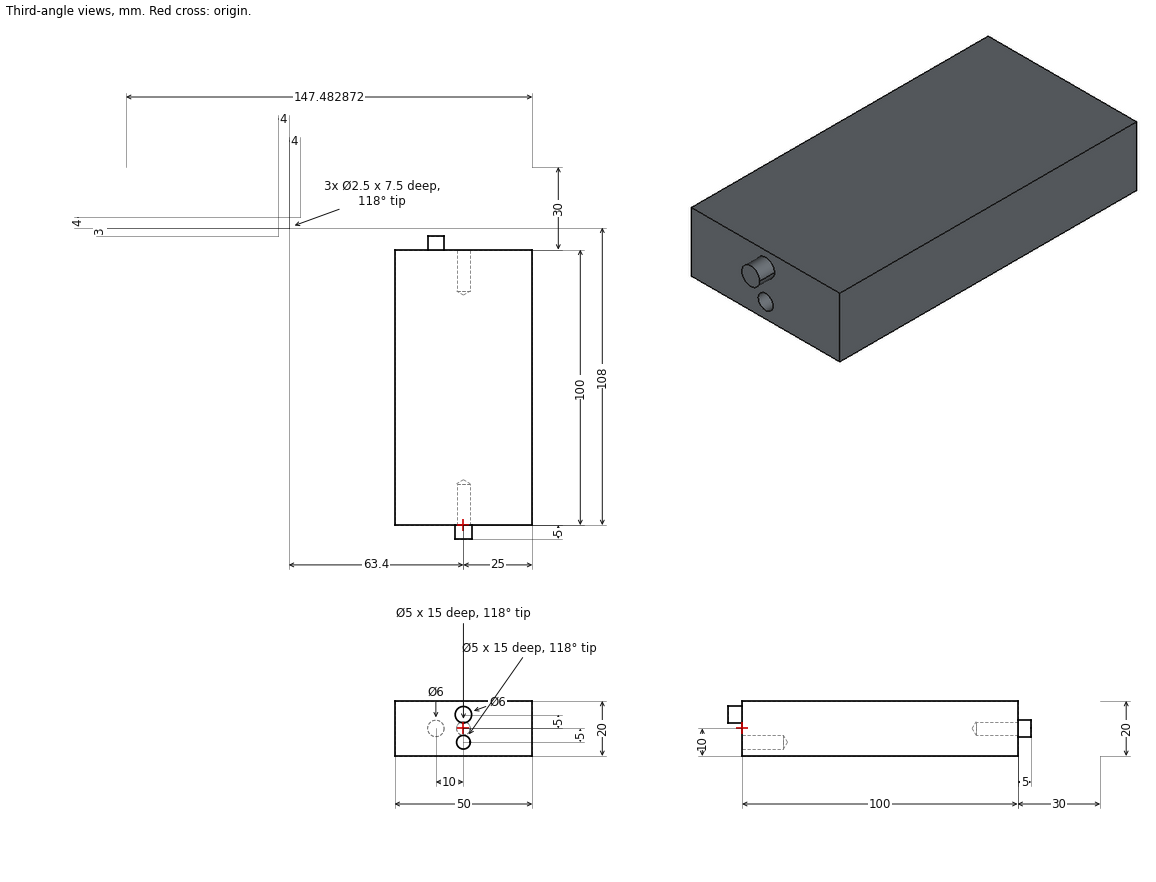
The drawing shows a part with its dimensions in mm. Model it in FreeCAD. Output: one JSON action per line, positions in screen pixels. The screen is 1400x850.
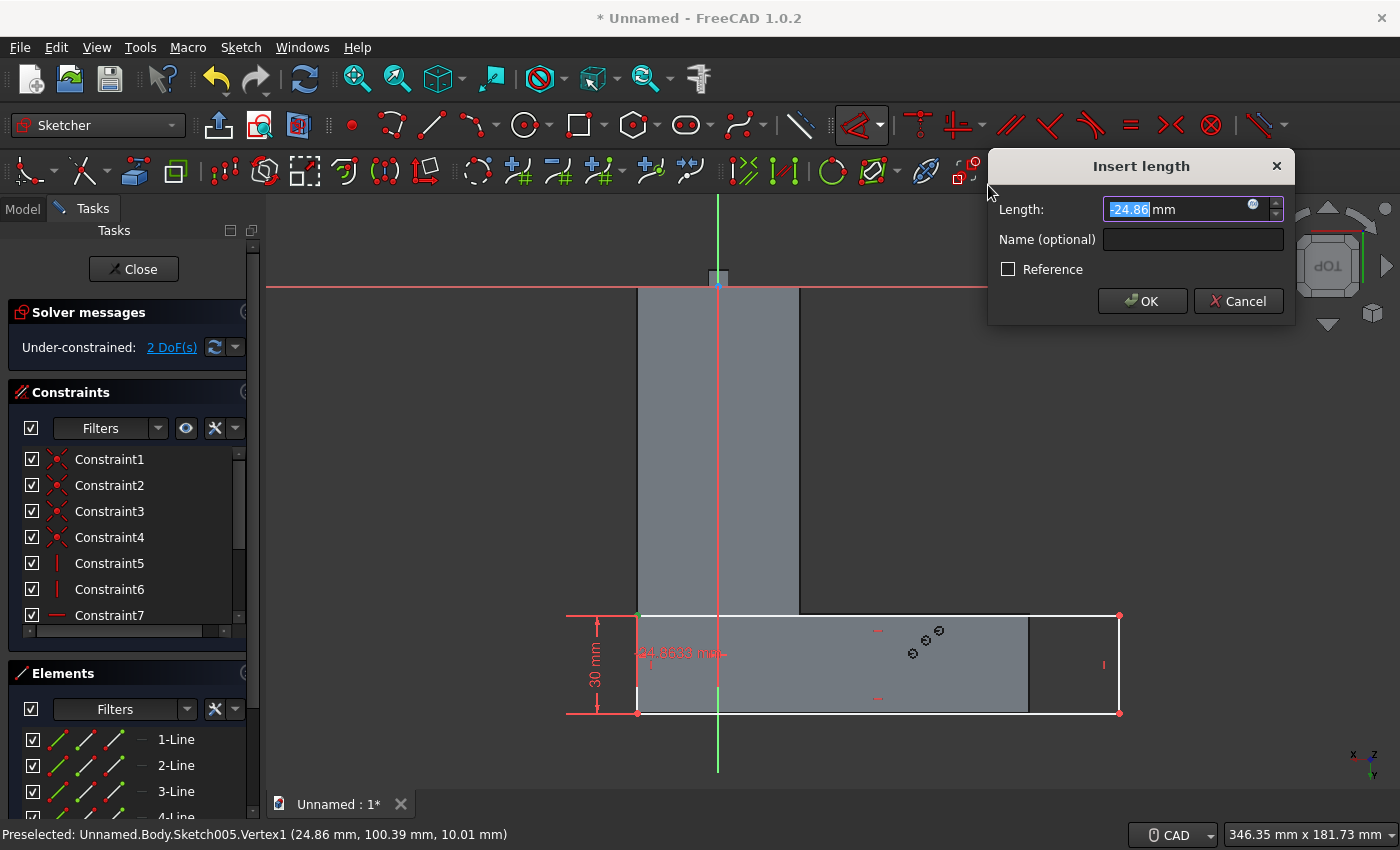
{"action": "type", "text": "-25"}
{"action": "key", "text": "Return"}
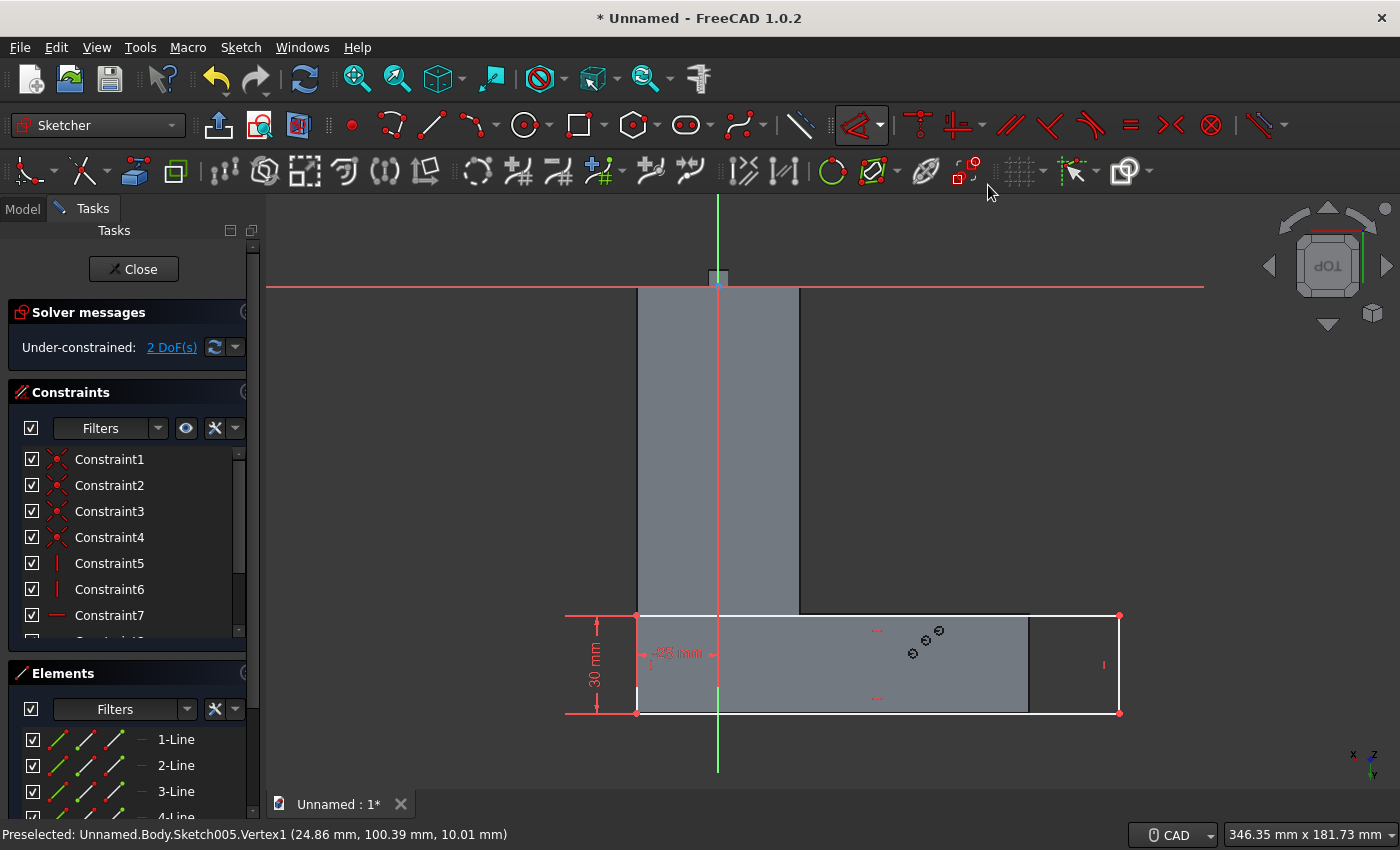
{"action": "left_click", "coordinate": [637, 616]}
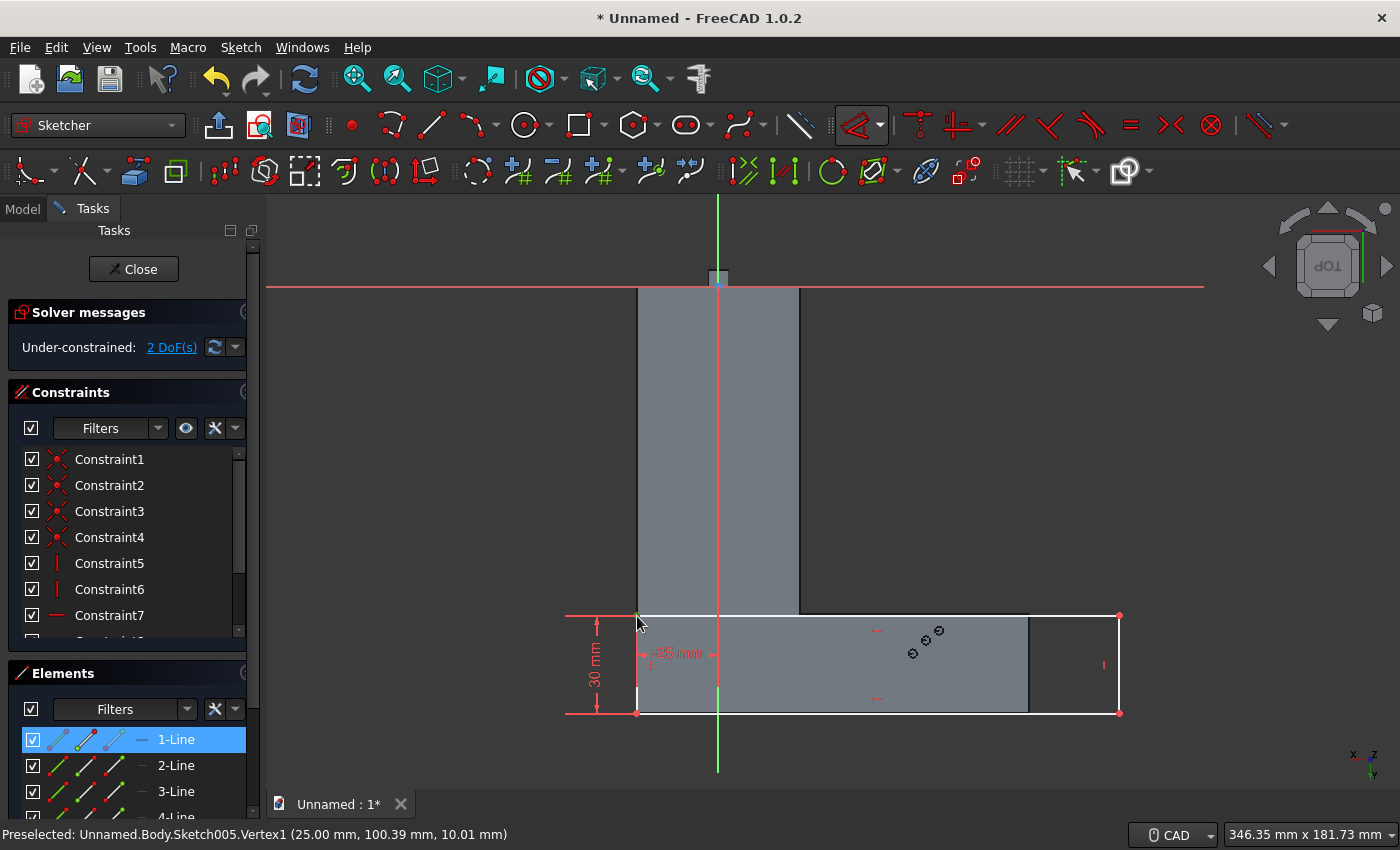
{"action": "key", "text": "i"}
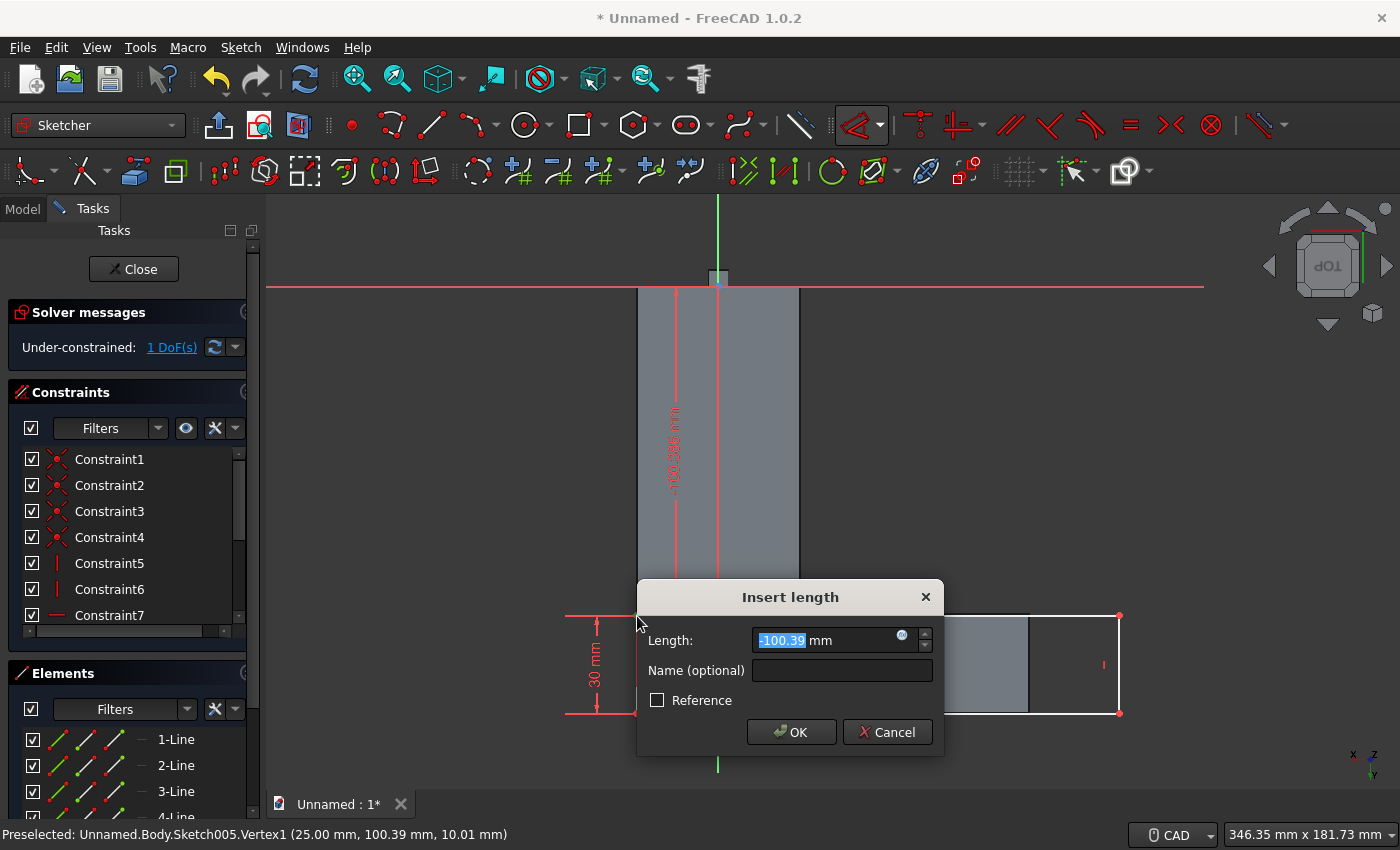
{"action": "type", "text": "-100"}
{"action": "key", "text": "Return"}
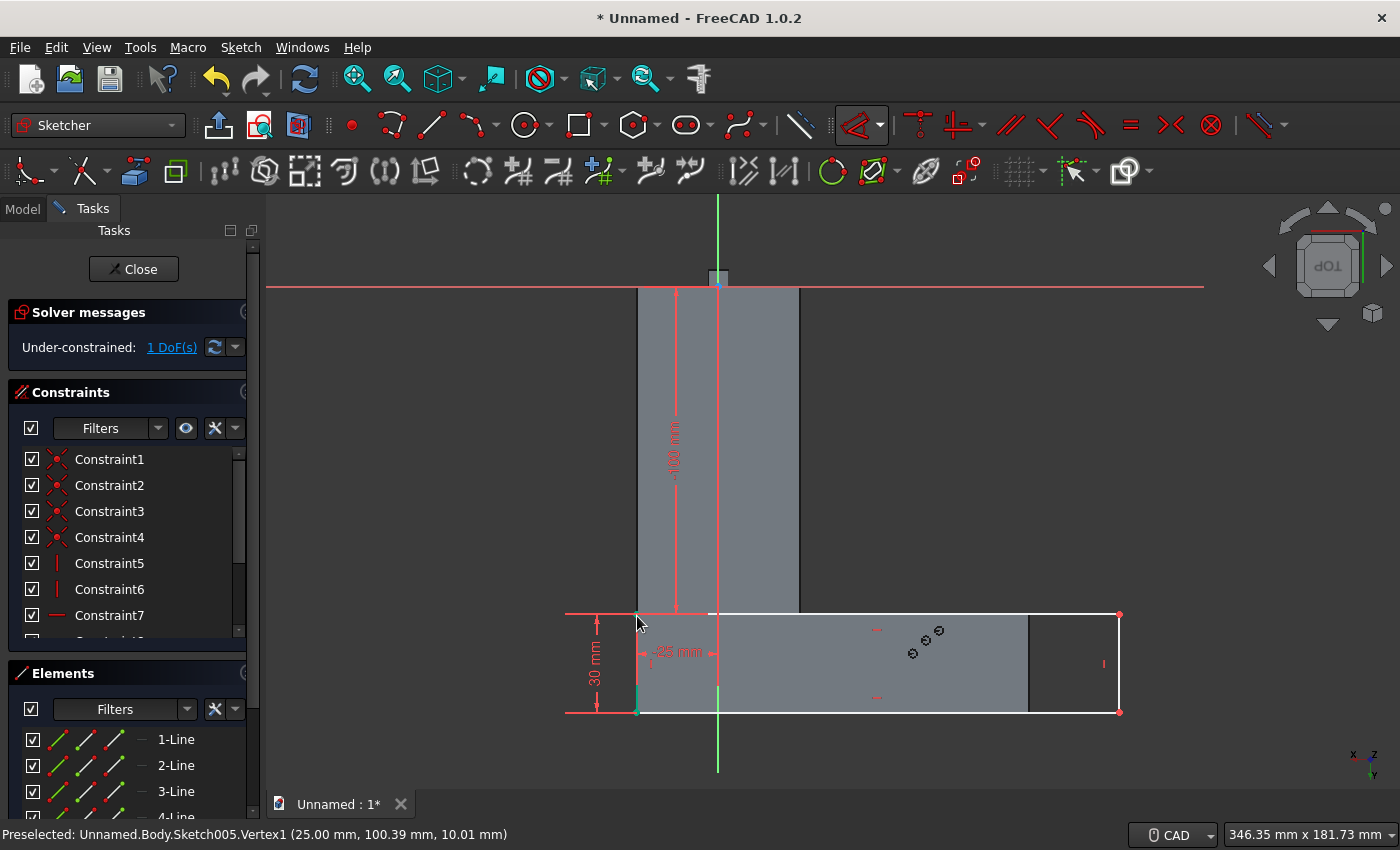
{"action": "left_click", "coordinate": [781, 713]}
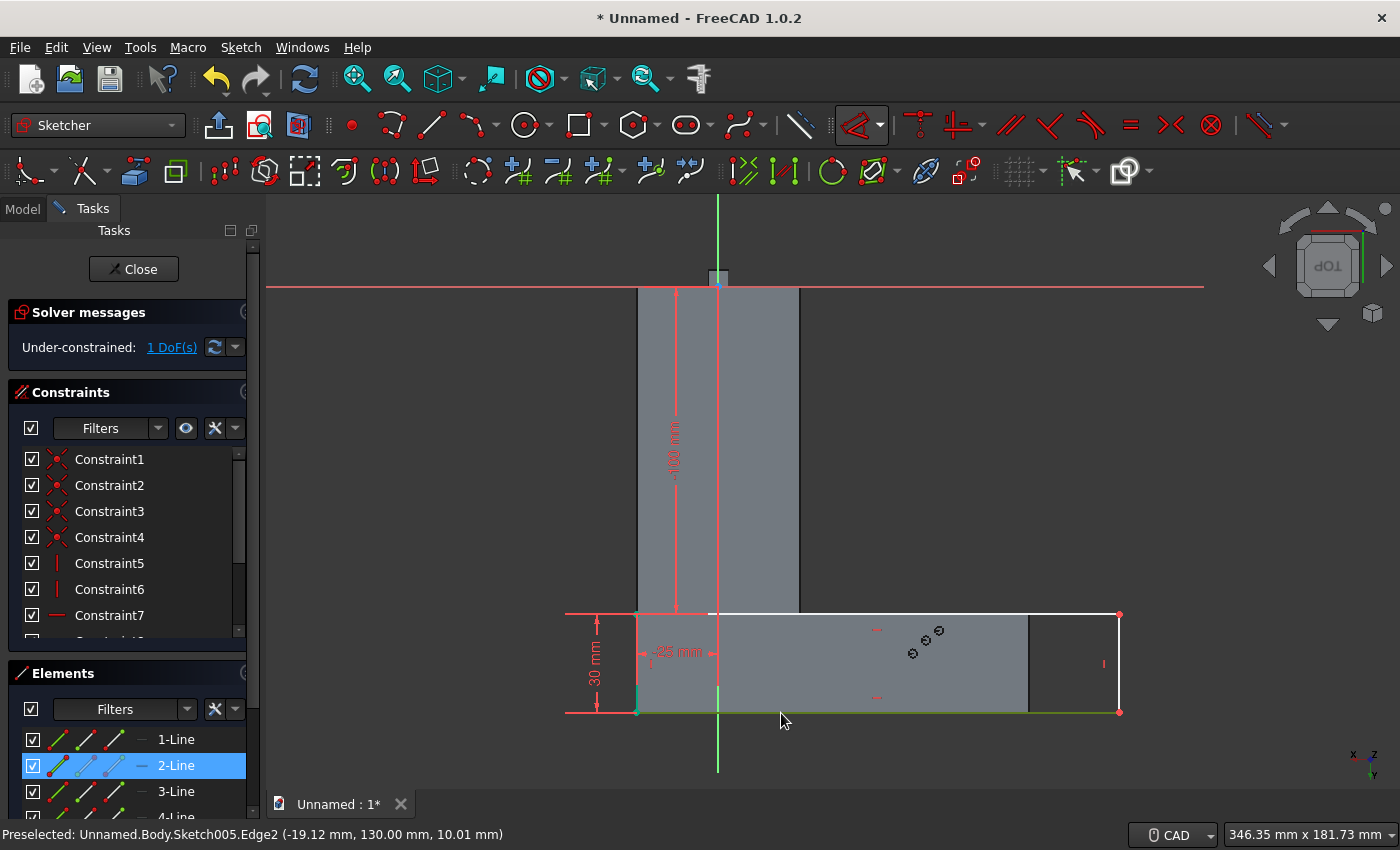
{"action": "key", "text": "l"}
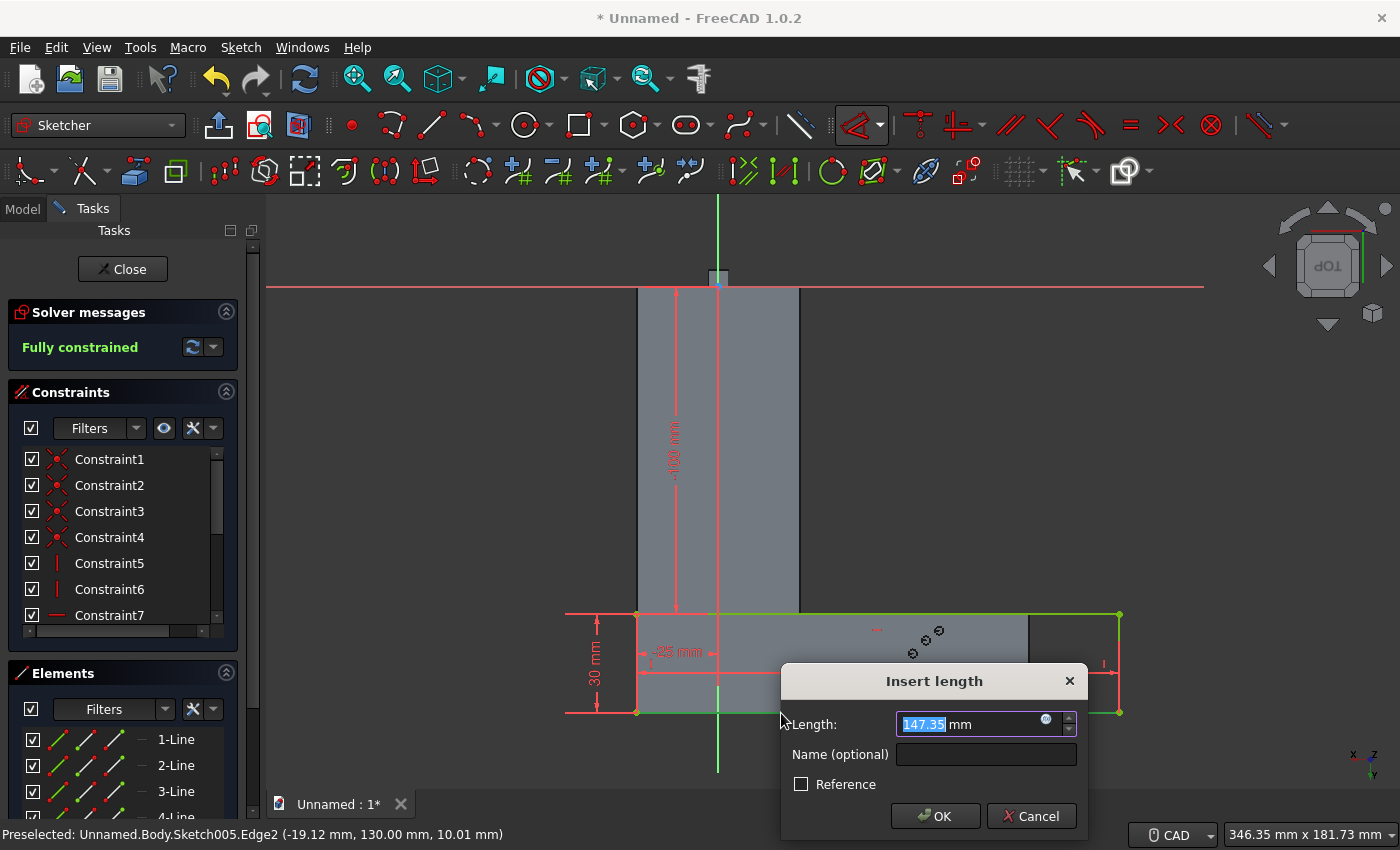
{"action": "type", "text": "147.482872"}
{"action": "key", "text": "Return"}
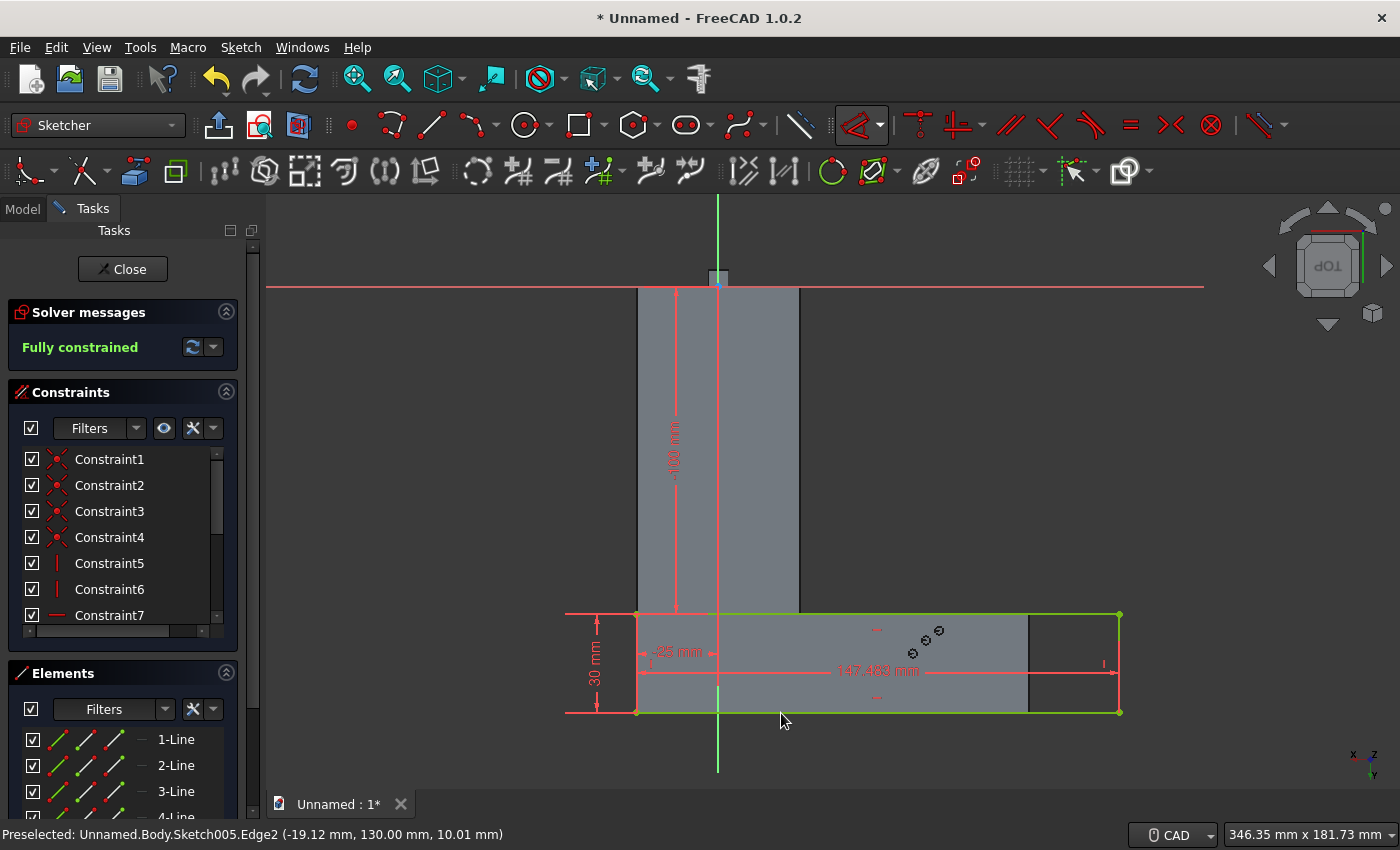
{"action": "left_click", "coordinate": [123, 269]}